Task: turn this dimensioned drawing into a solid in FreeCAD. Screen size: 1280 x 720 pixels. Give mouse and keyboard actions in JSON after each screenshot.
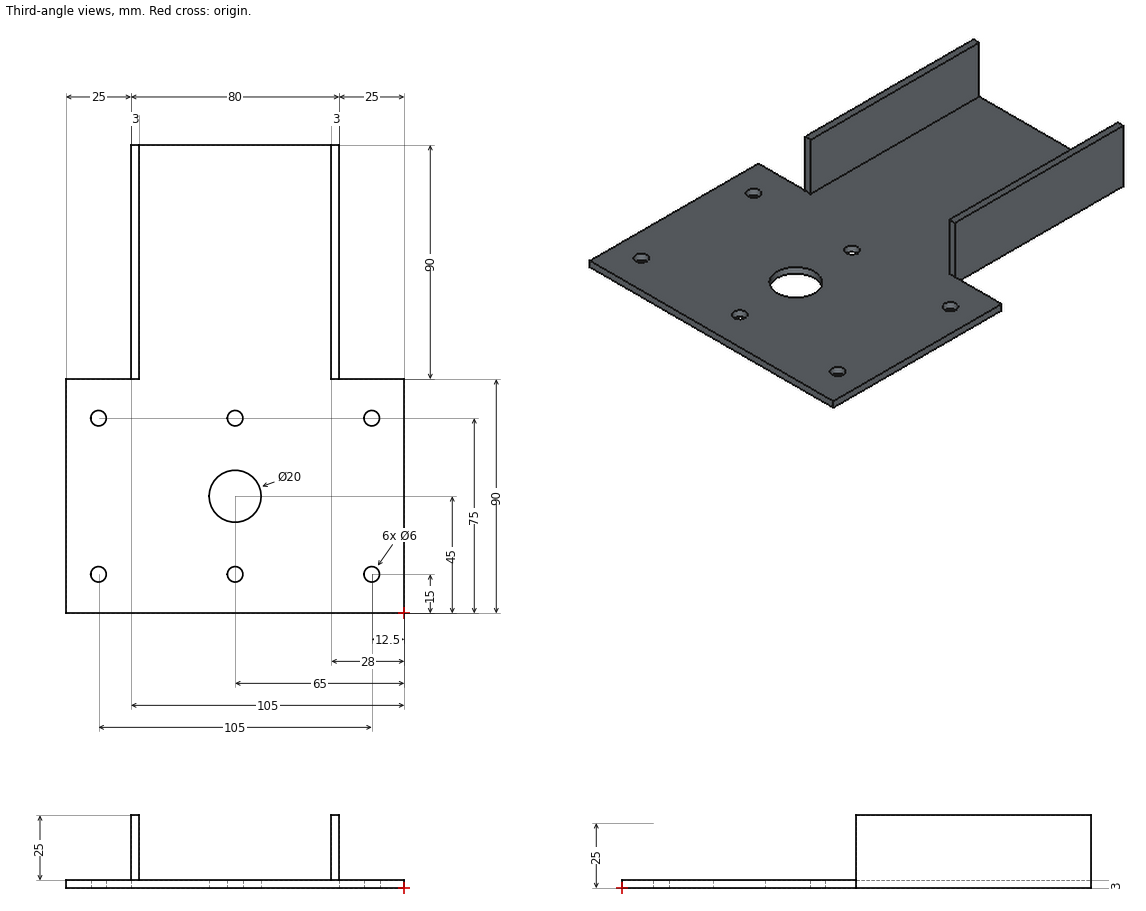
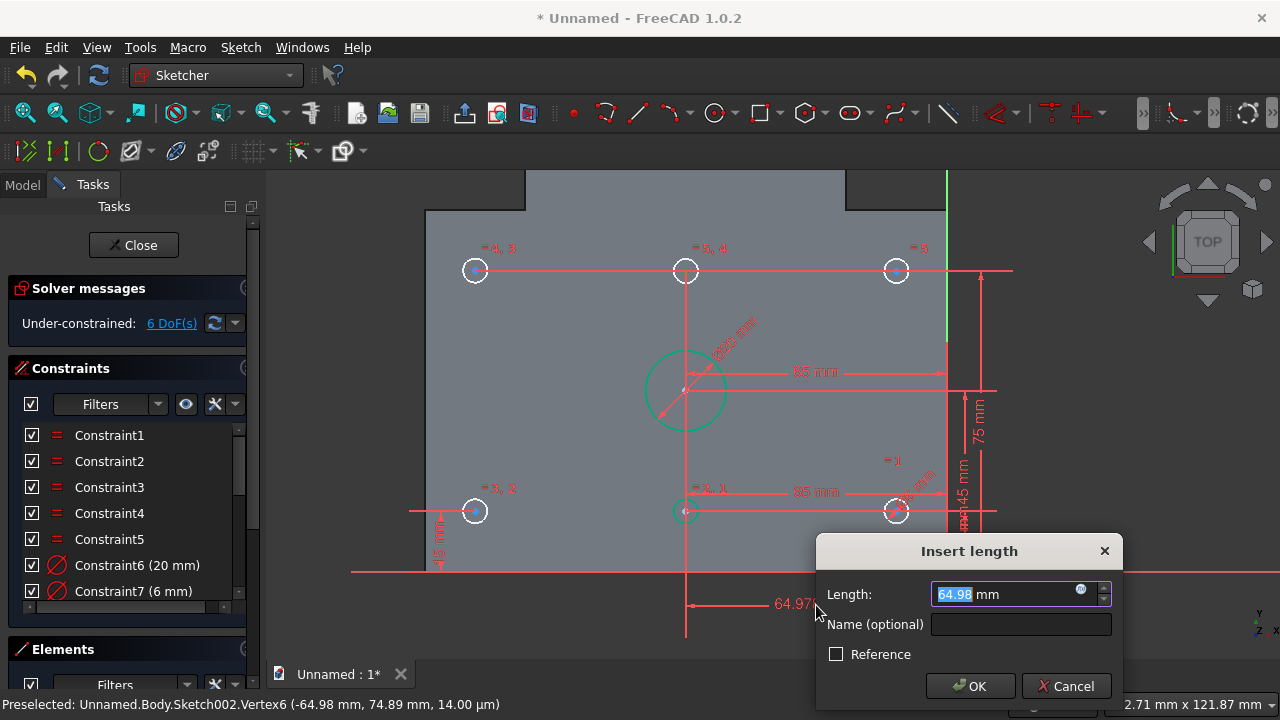
{"action": "type", "text": "65"}
{"action": "key", "text": "Return"}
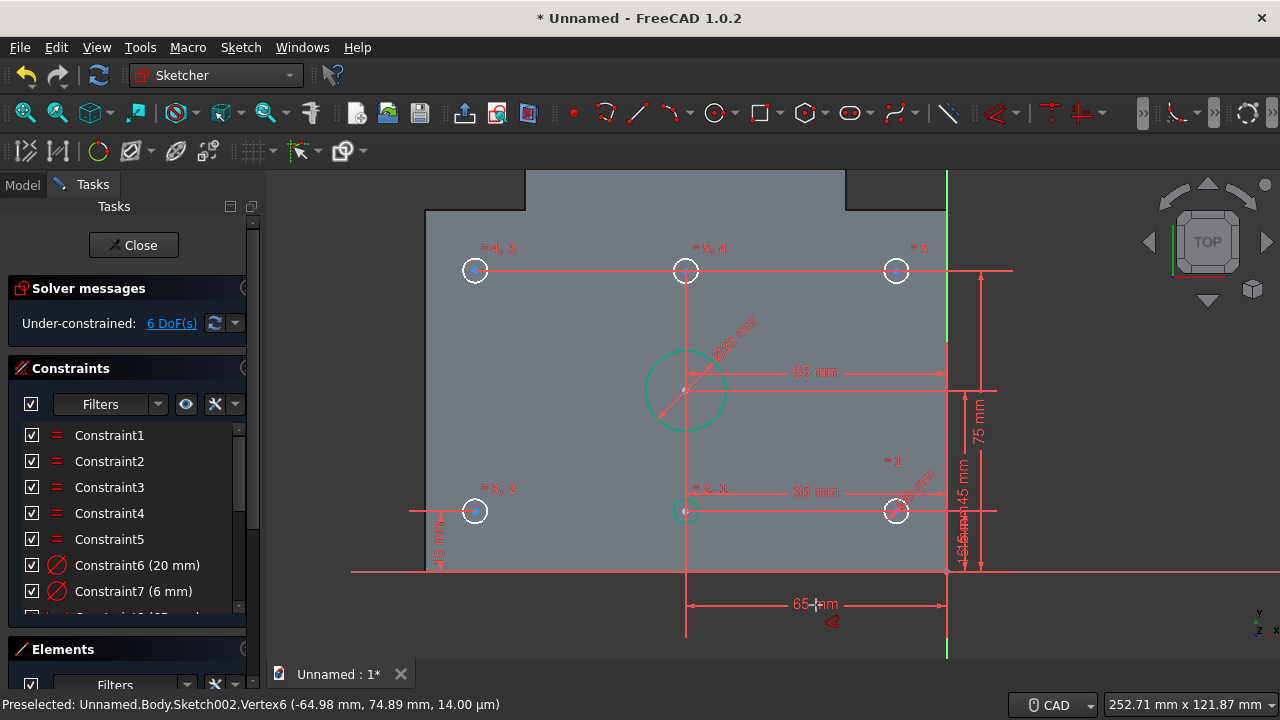
{"action": "left_click", "coordinate": [686, 271]}
{"action": "left_click", "coordinate": [981, 352]}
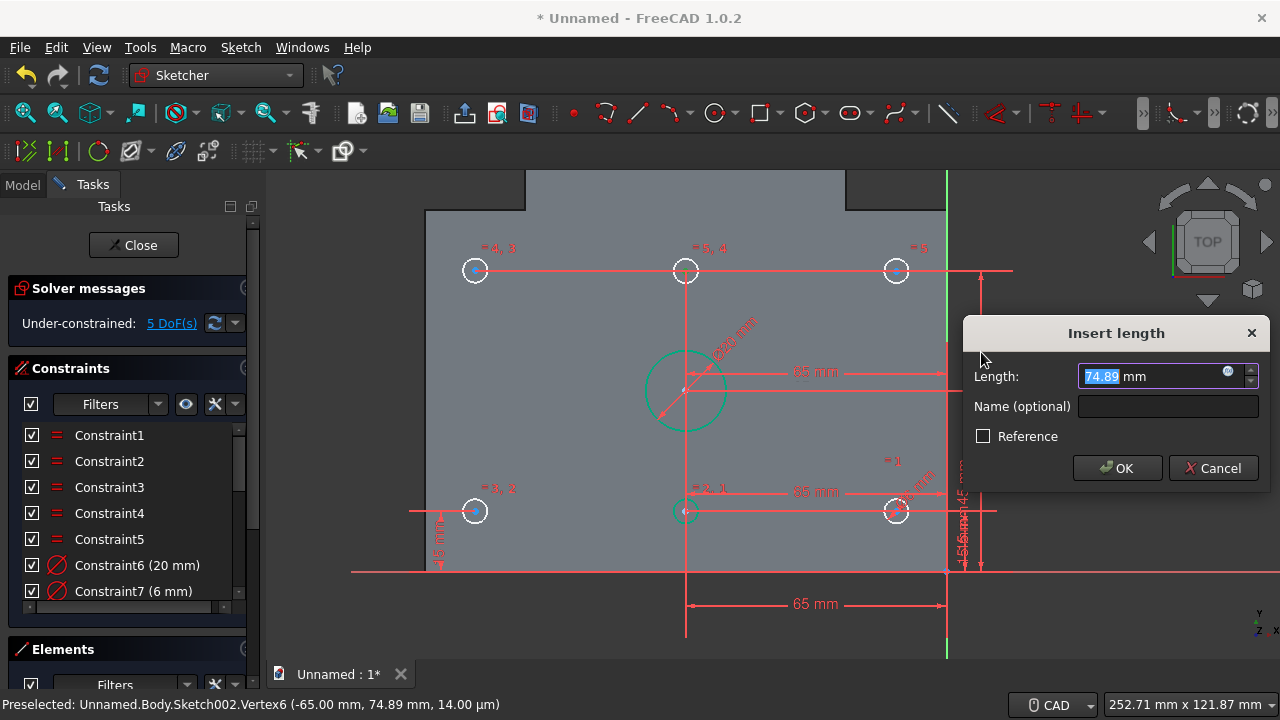
{"action": "type", "text": "75"}
{"action": "key", "text": "Return"}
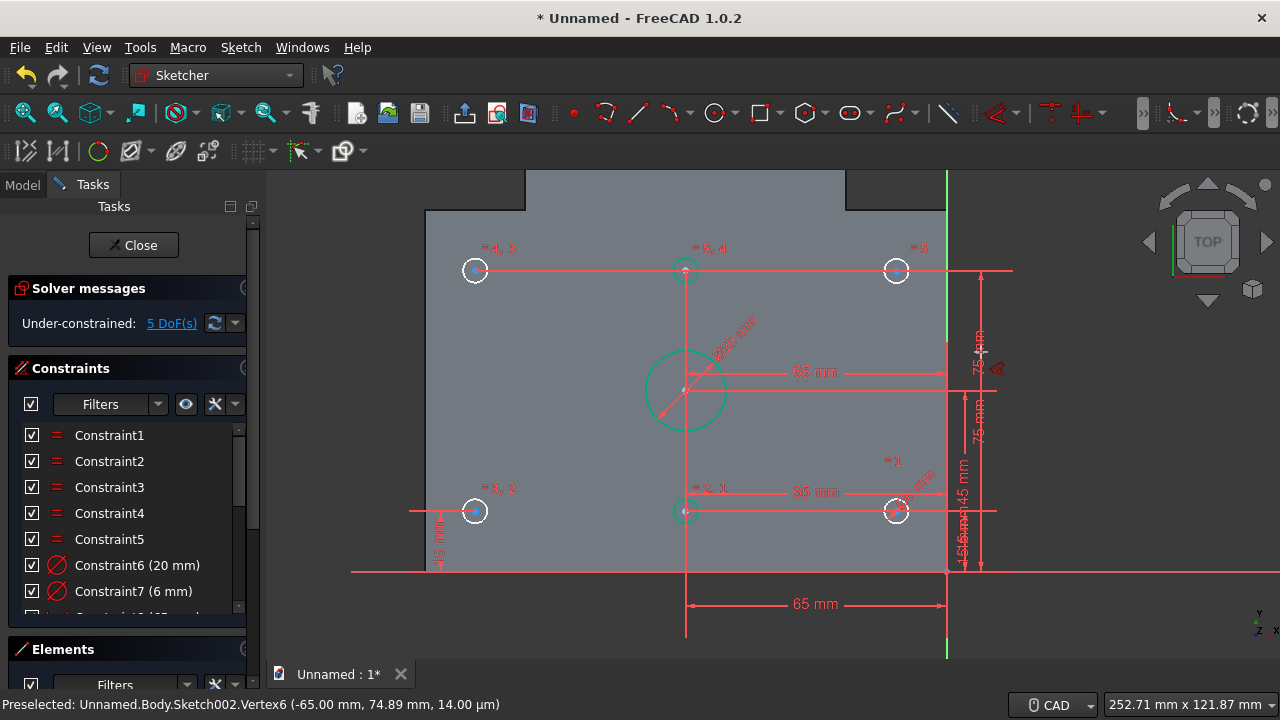
{"action": "left_click", "coordinate": [896, 271]}
{"action": "left_click", "coordinate": [981, 316]}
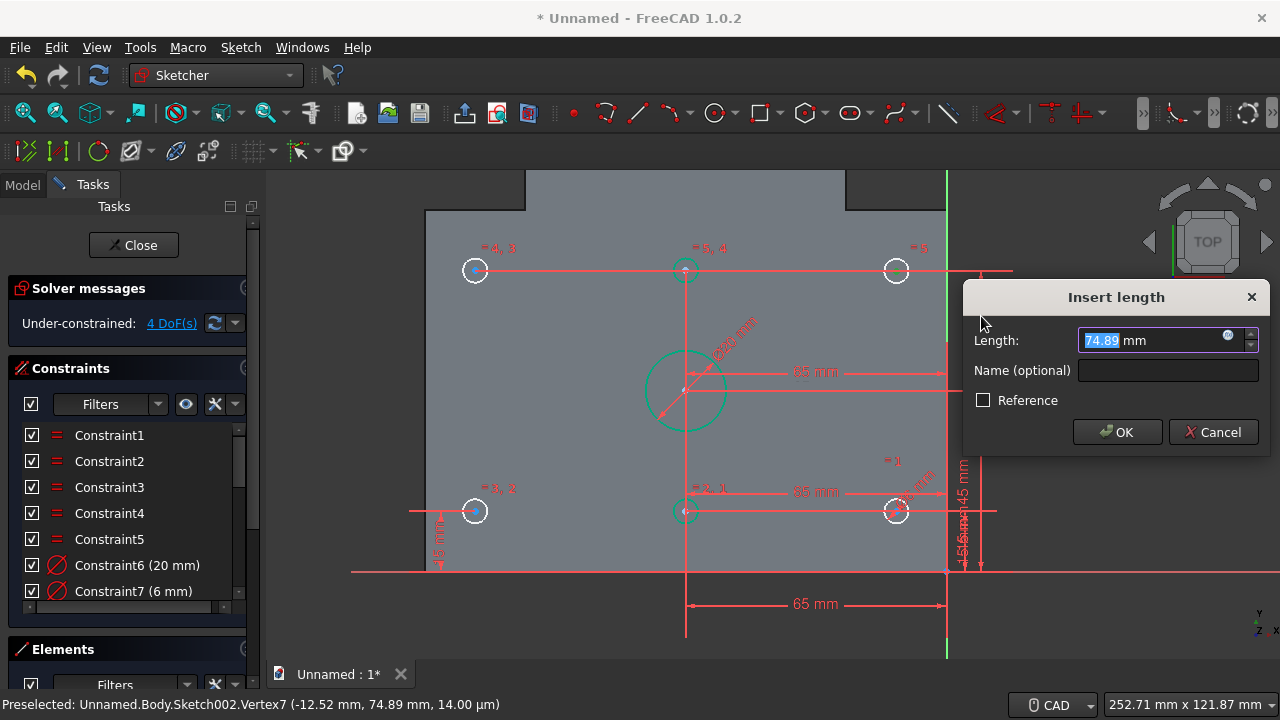
{"action": "type", "text": "75"}
{"action": "key", "text": "Return"}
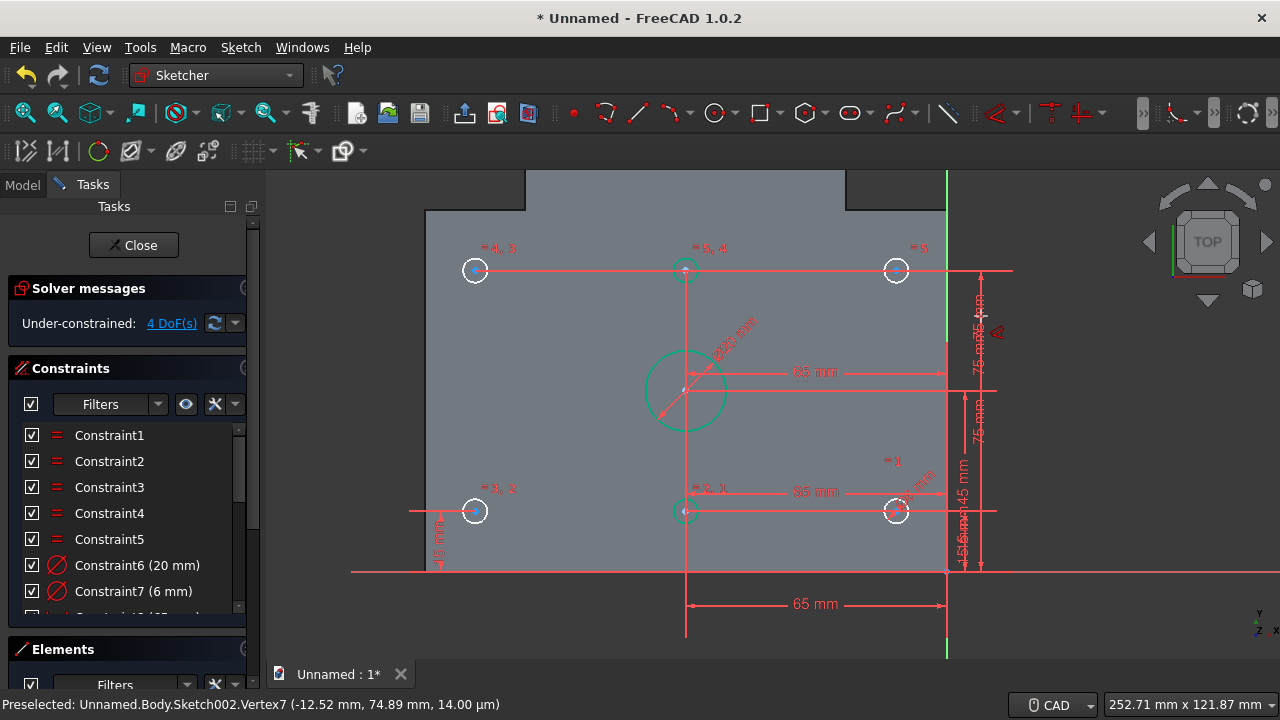
{"action": "left_click", "coordinate": [896, 511]}
{"action": "left_click", "coordinate": [922, 605]}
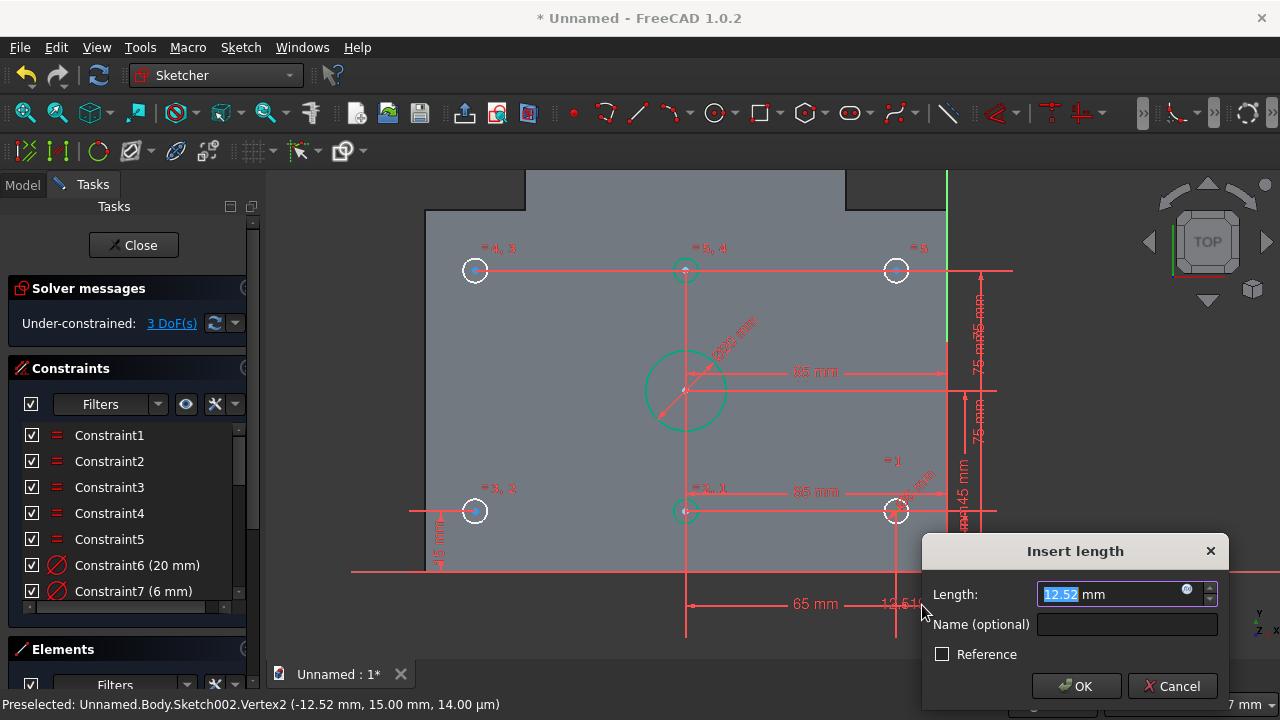
{"action": "type", "text": "12.5"}
{"action": "key", "text": "Return"}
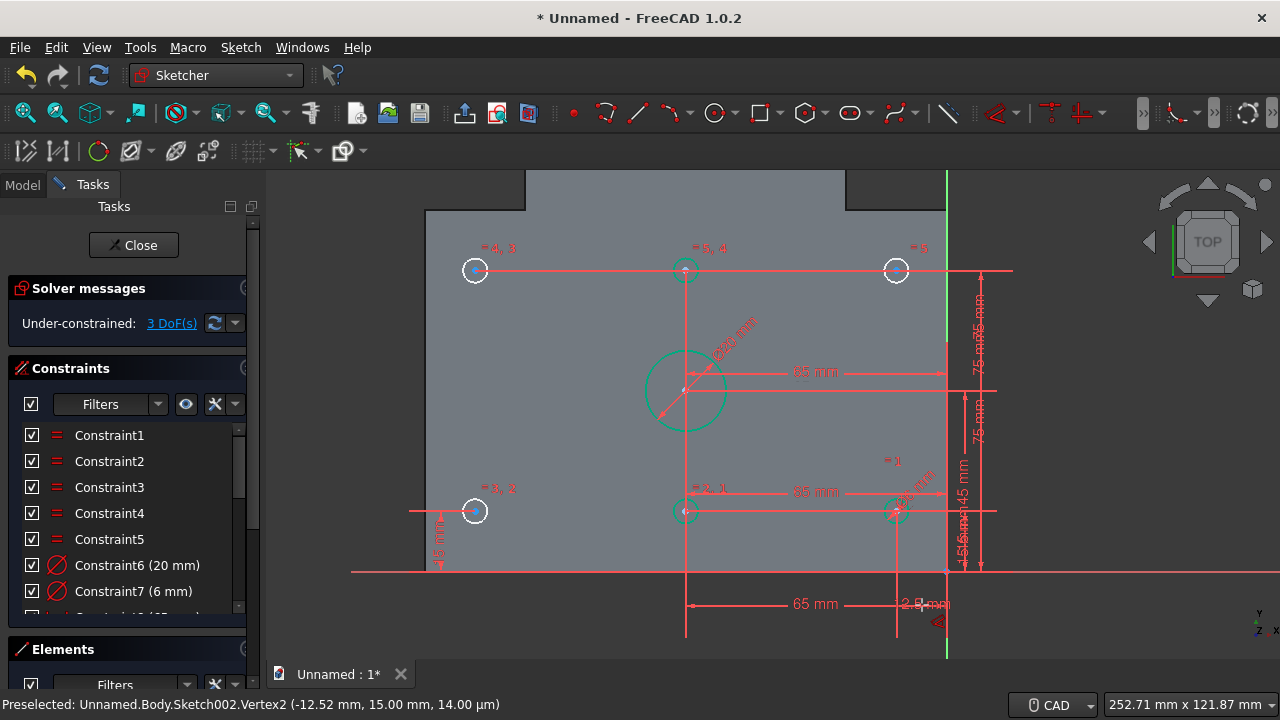
{"action": "left_click", "coordinate": [896, 271]}
{"action": "left_click", "coordinate": [922, 237]}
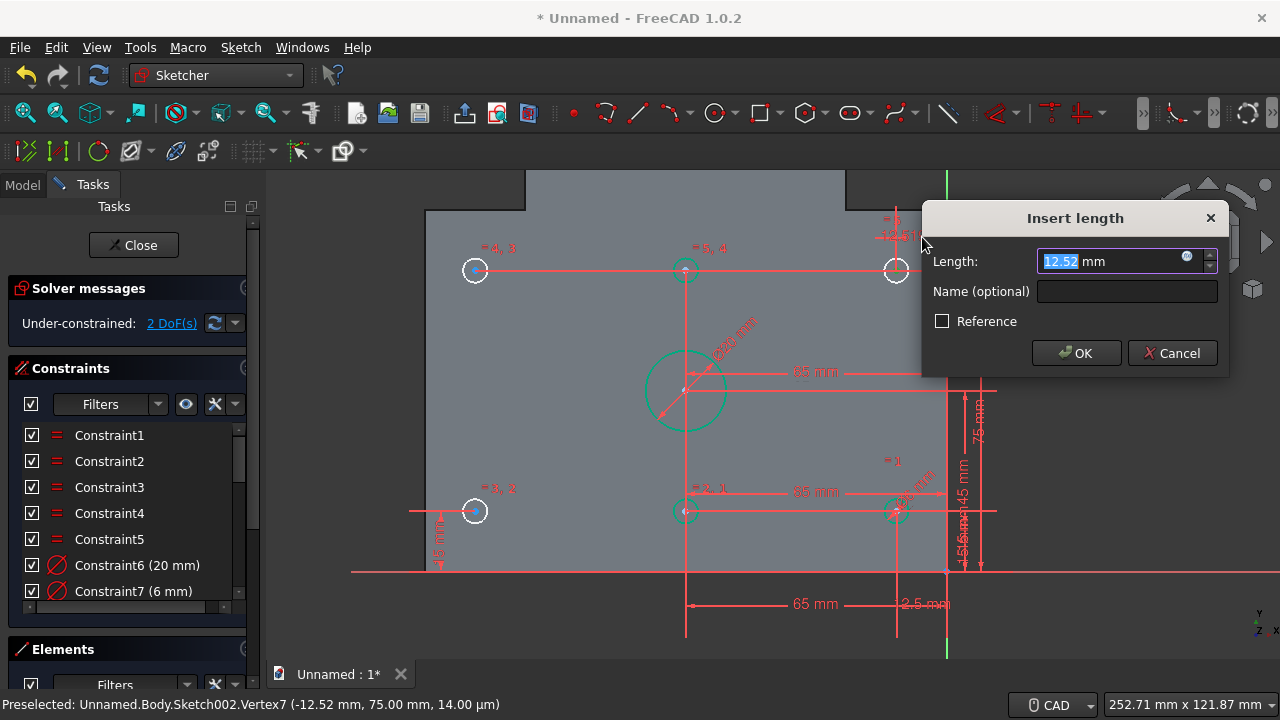
{"action": "type", "text": "12.5"}
{"action": "key", "text": "Return"}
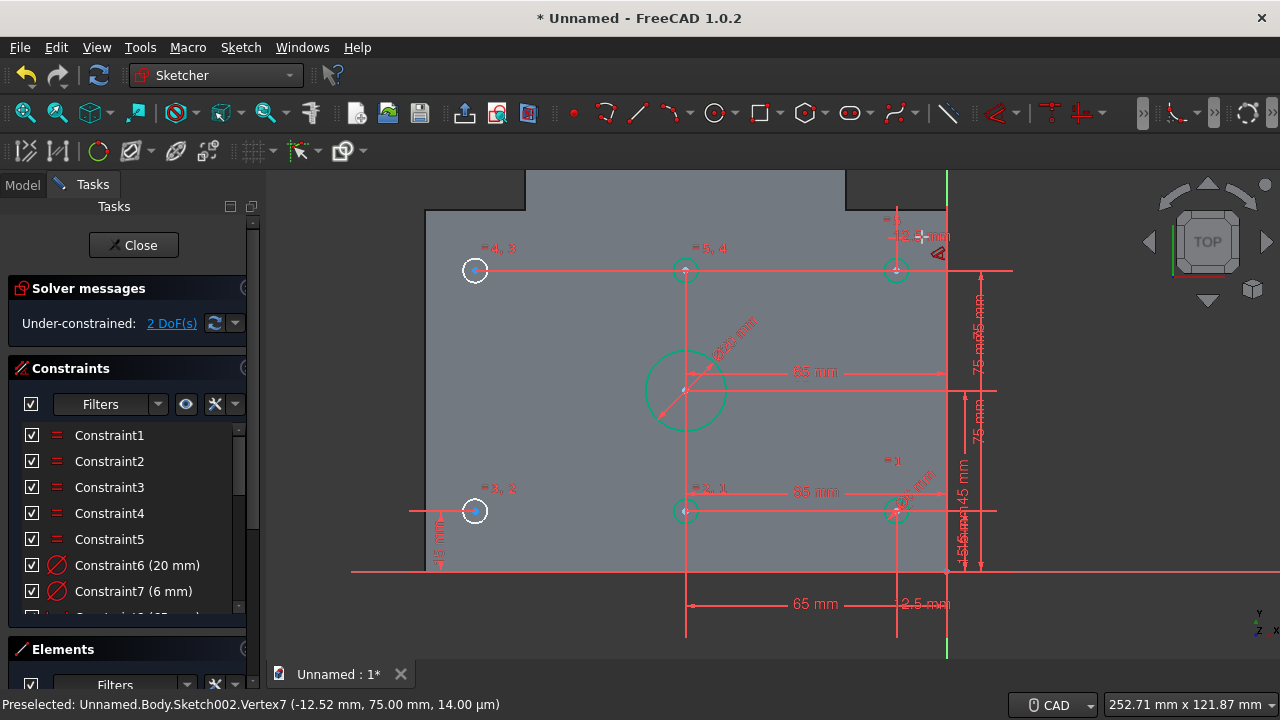
{"action": "left_click", "coordinate": [897, 511]}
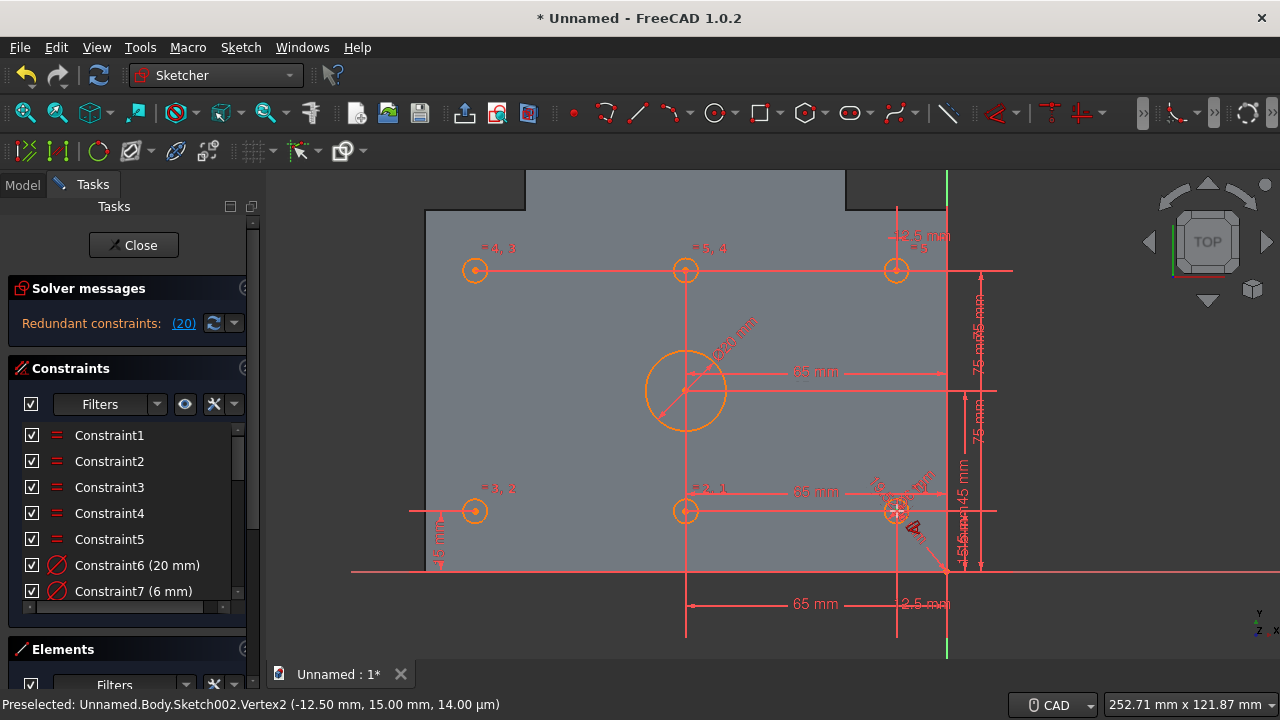
{"action": "left_click", "coordinate": [475, 511]}
{"action": "left_click", "coordinate": [686, 545]}